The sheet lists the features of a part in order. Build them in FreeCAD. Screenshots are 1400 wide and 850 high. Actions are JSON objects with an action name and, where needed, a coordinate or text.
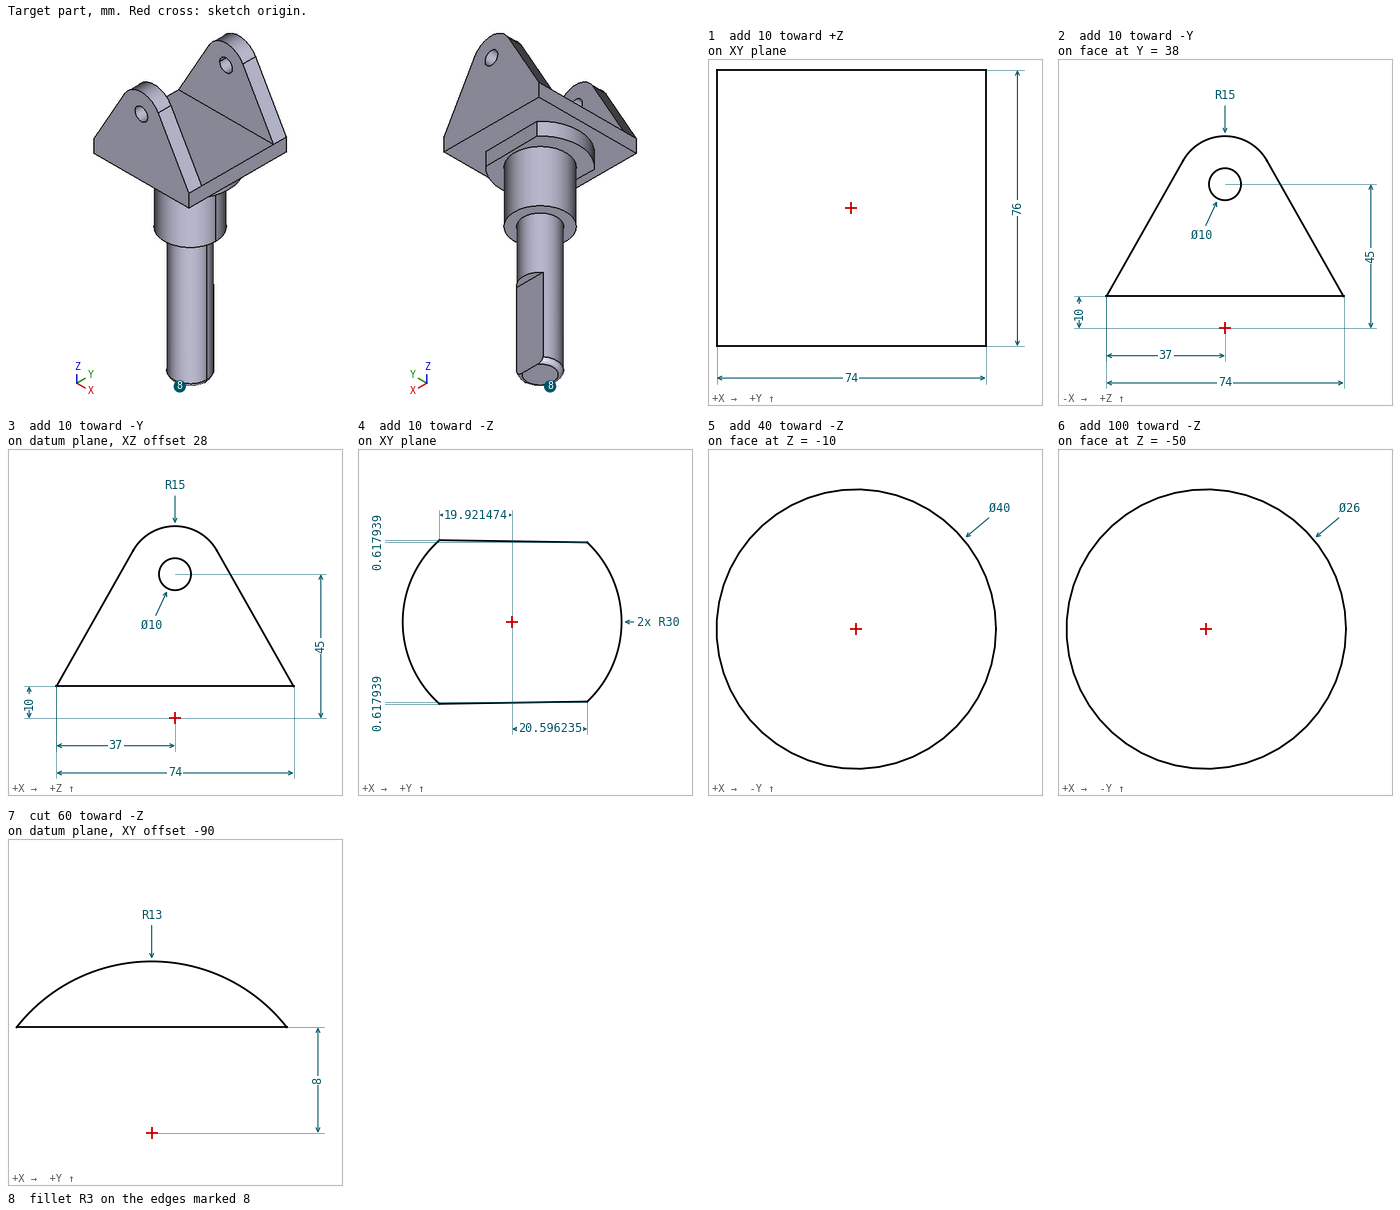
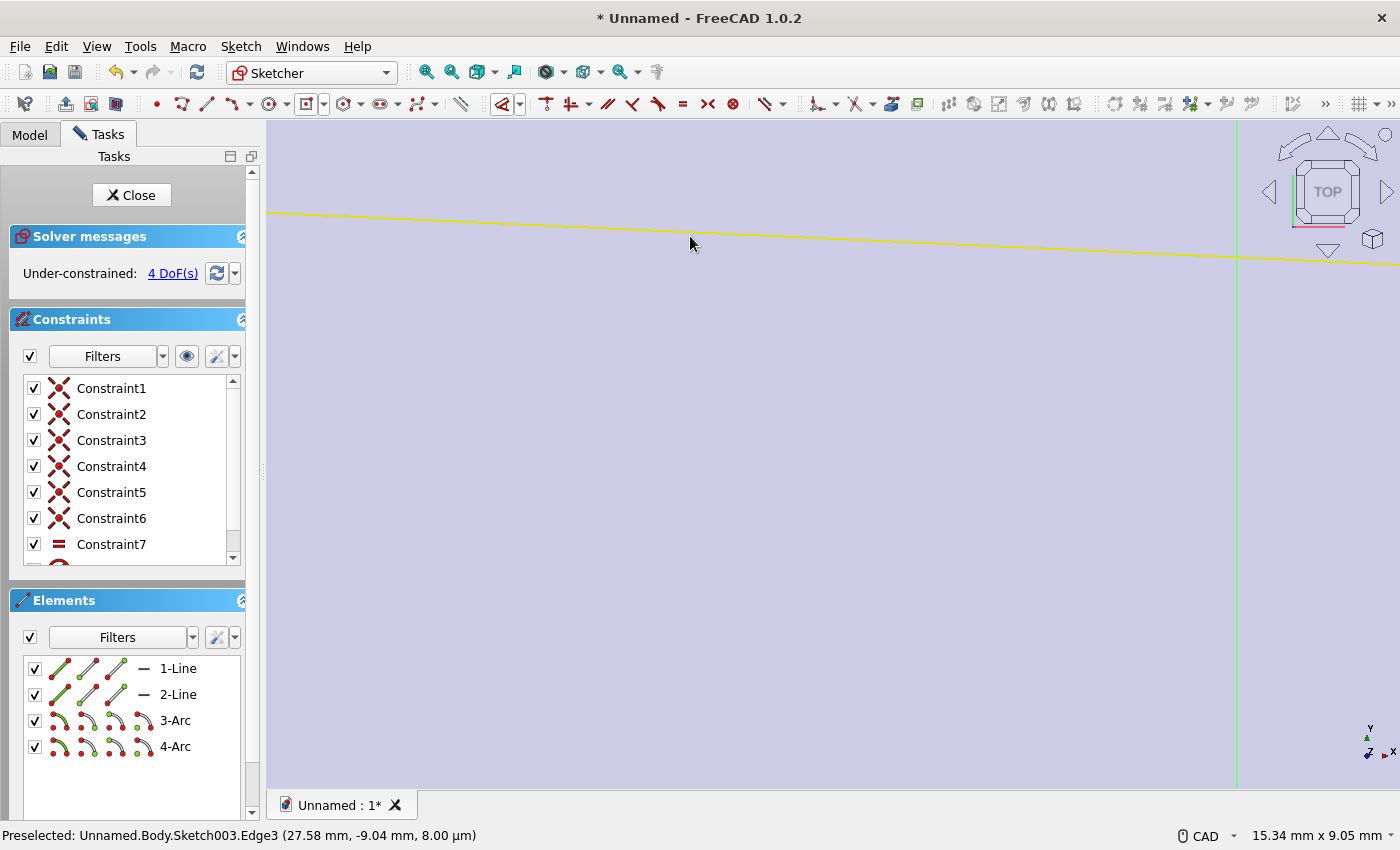
{"action": "left_click", "coordinate": [691, 232]}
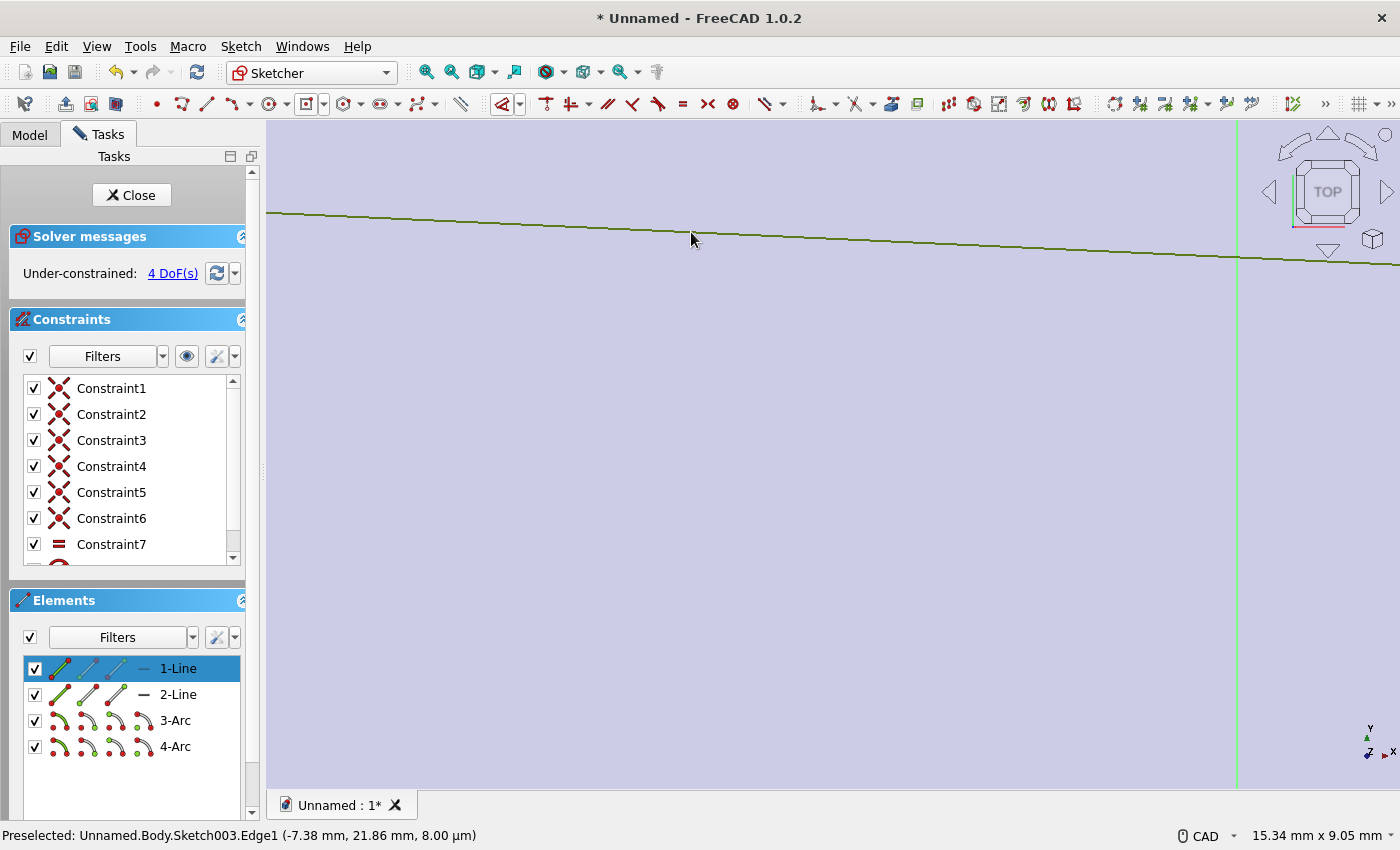
{"action": "left_click", "coordinate": [520, 104]}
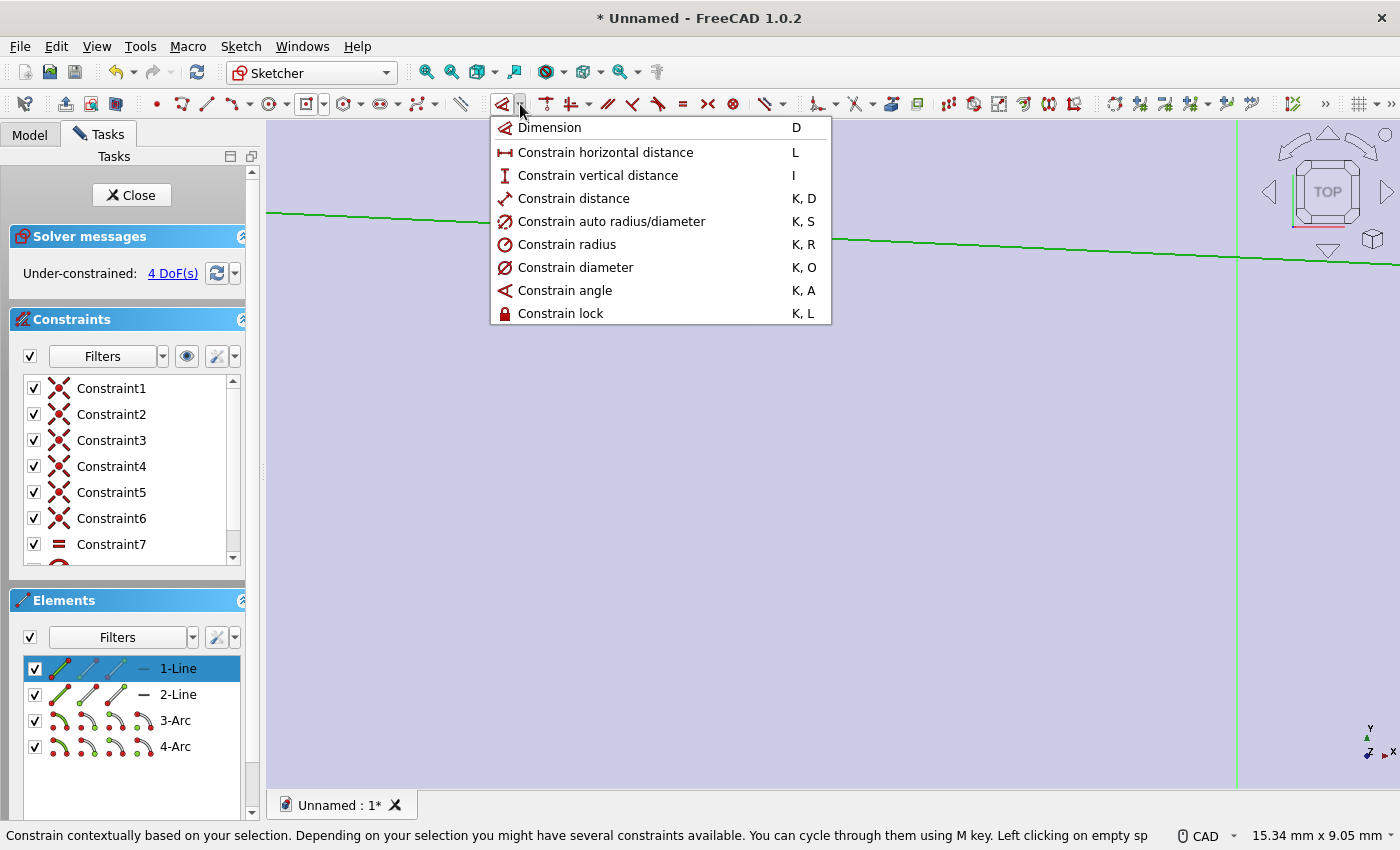
{"action": "left_click", "coordinate": [661, 176]}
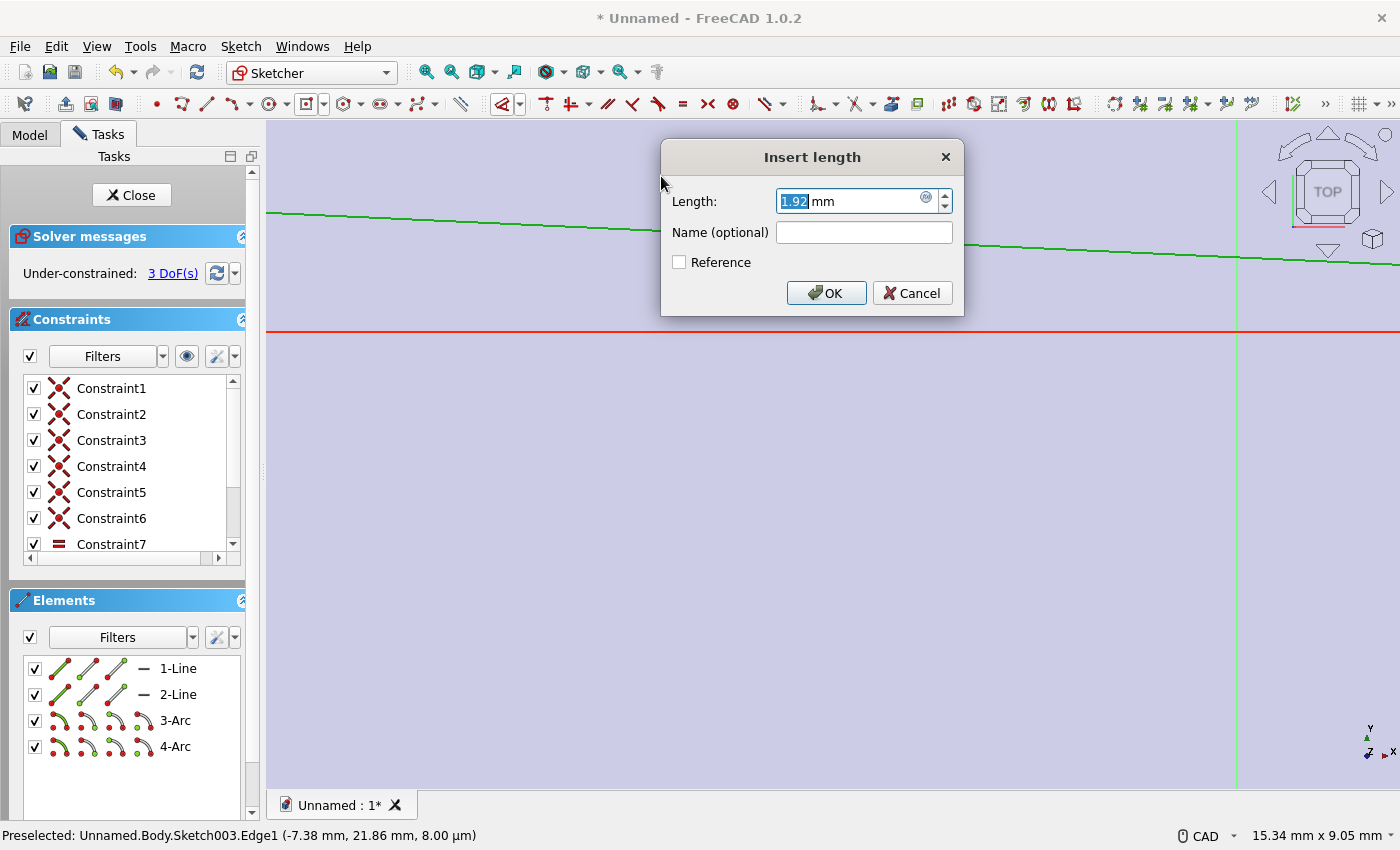
{"action": "type", "text": "0.617939"}
{"action": "key", "text": "Return"}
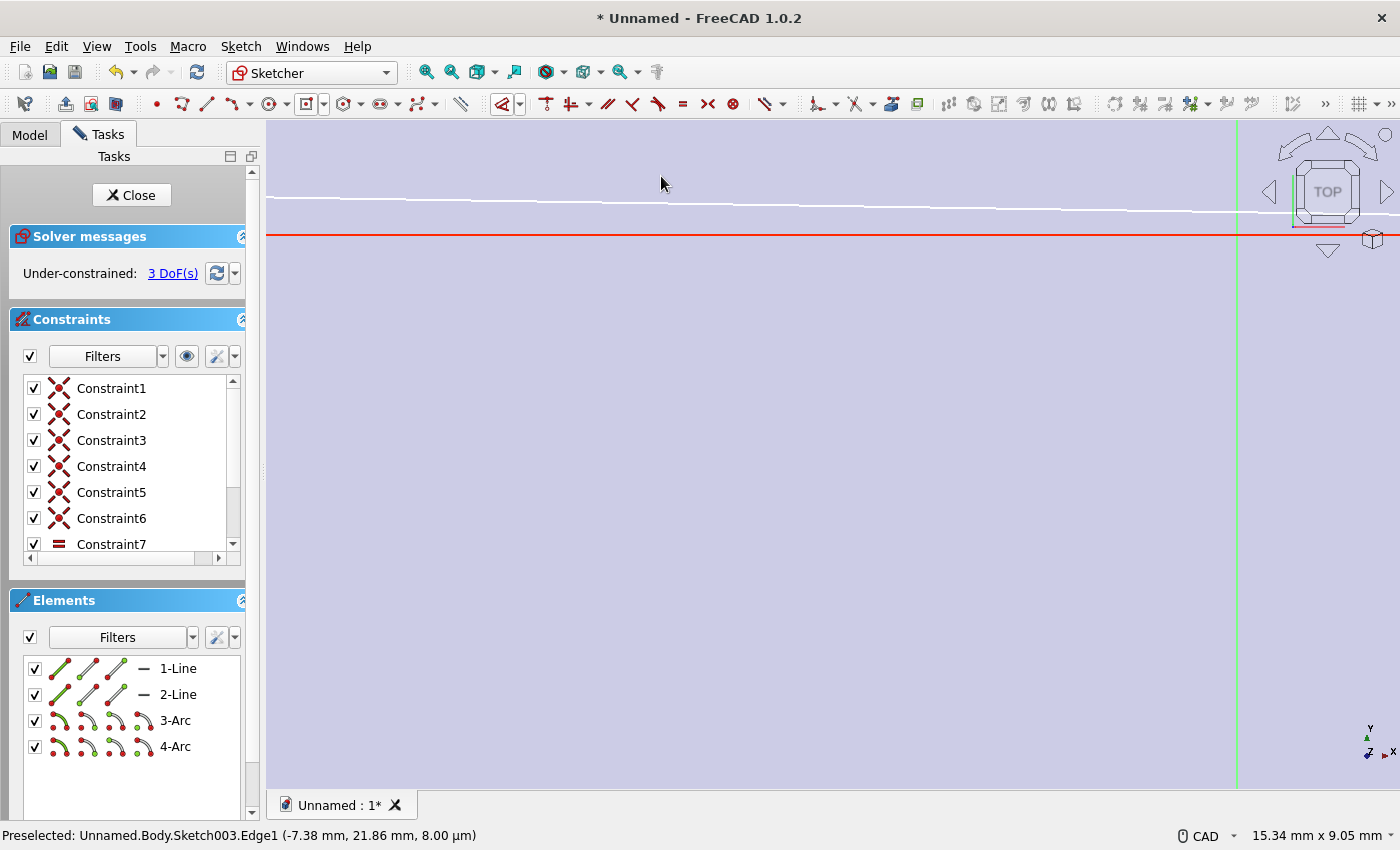
{"action": "scroll", "coordinate": [691, 236], "scroll_direction": "down", "scroll_amount": 10}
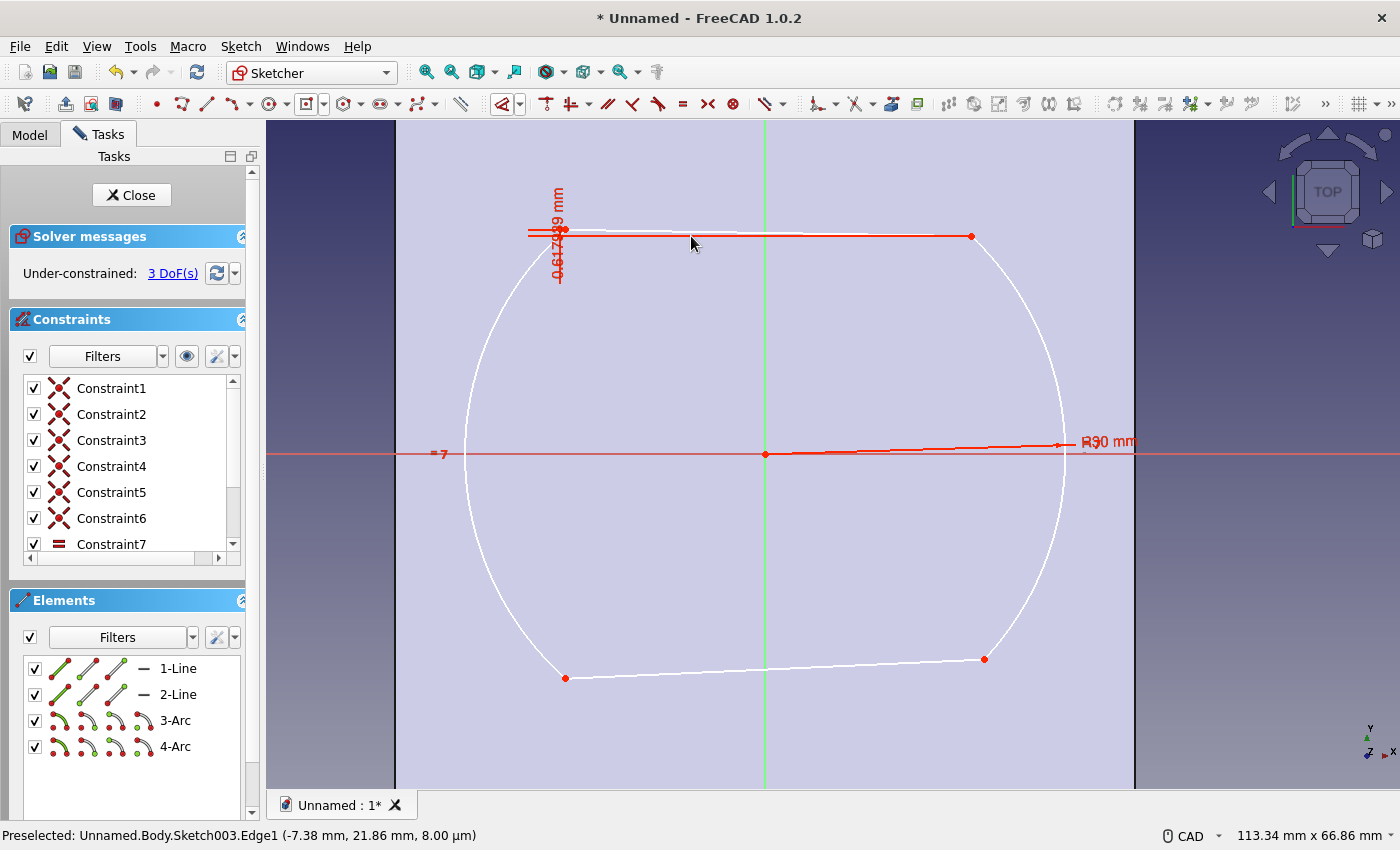
{"action": "scroll", "coordinate": [859, 665], "scroll_direction": "up", "scroll_amount": 10}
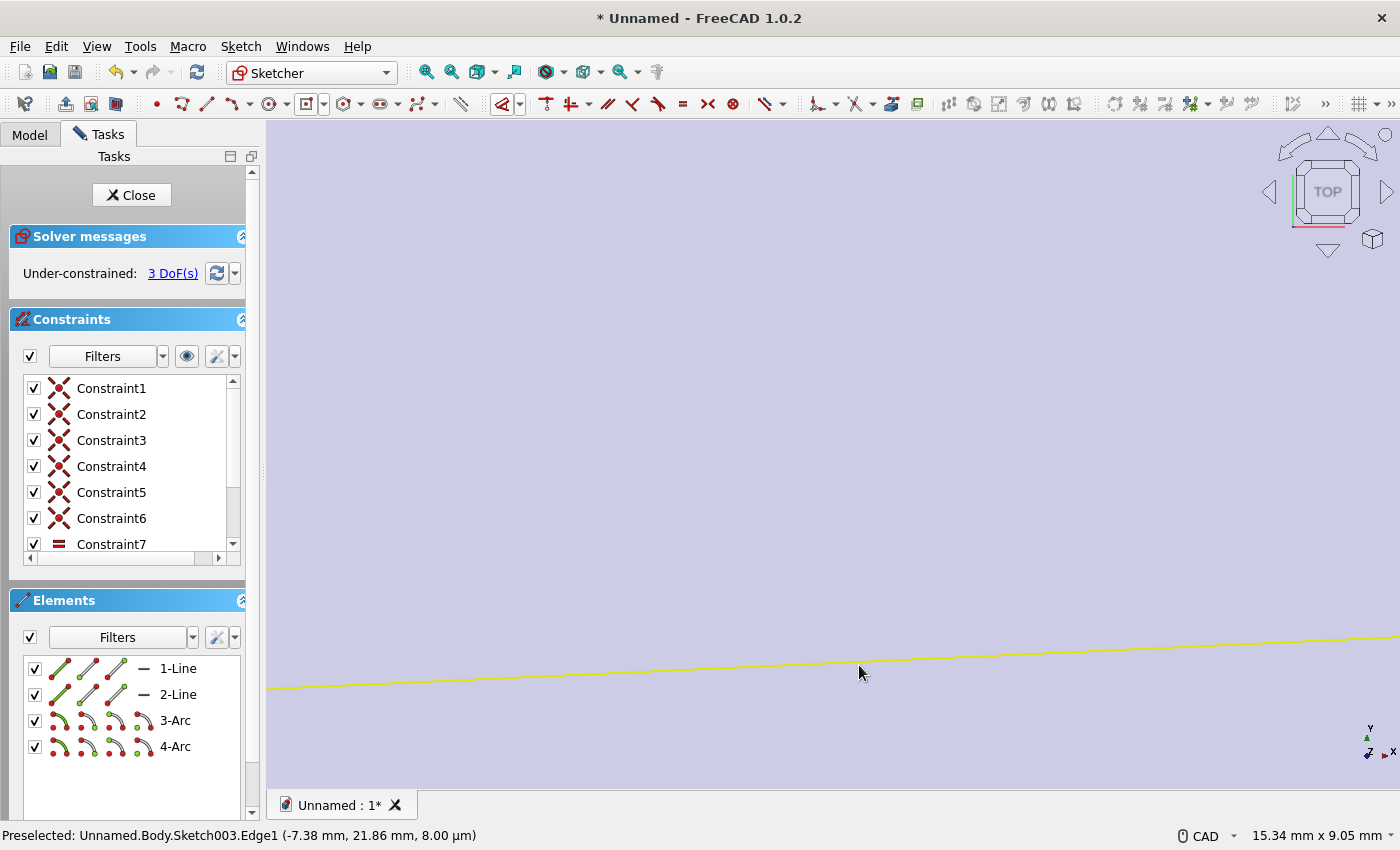
{"action": "left_click", "coordinate": [853, 662]}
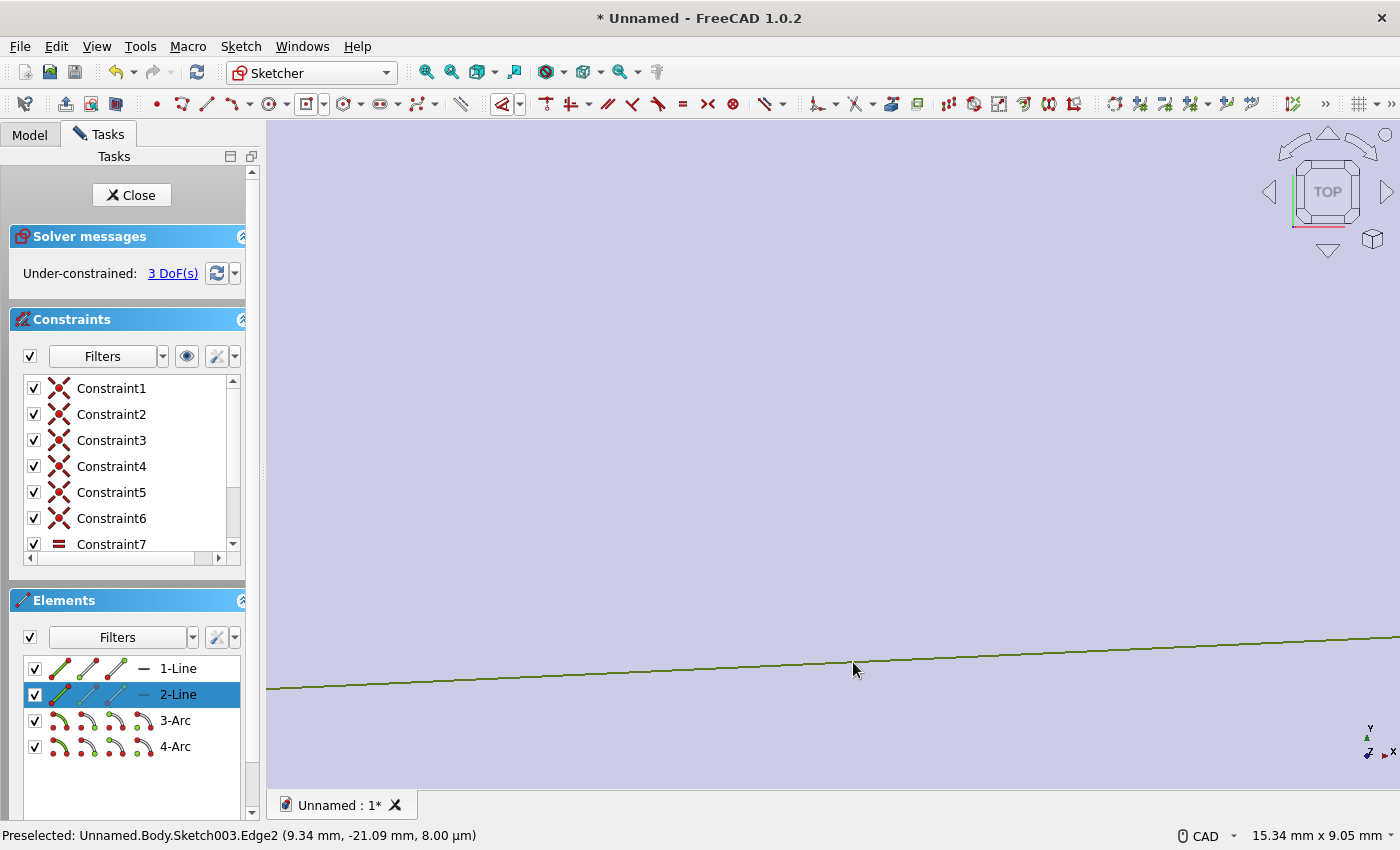
{"action": "left_click", "coordinate": [520, 104]}